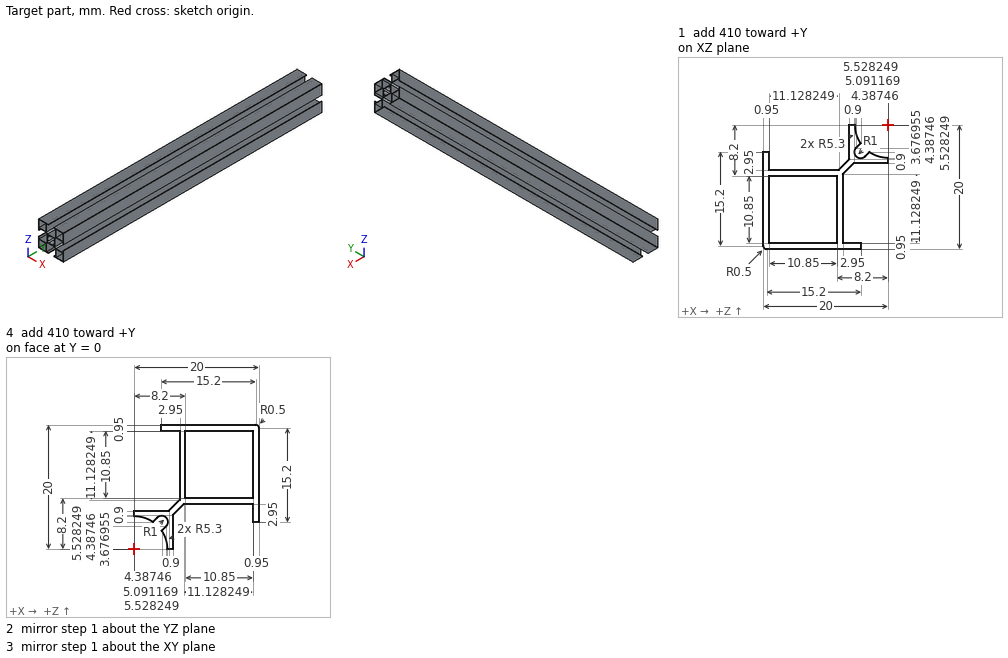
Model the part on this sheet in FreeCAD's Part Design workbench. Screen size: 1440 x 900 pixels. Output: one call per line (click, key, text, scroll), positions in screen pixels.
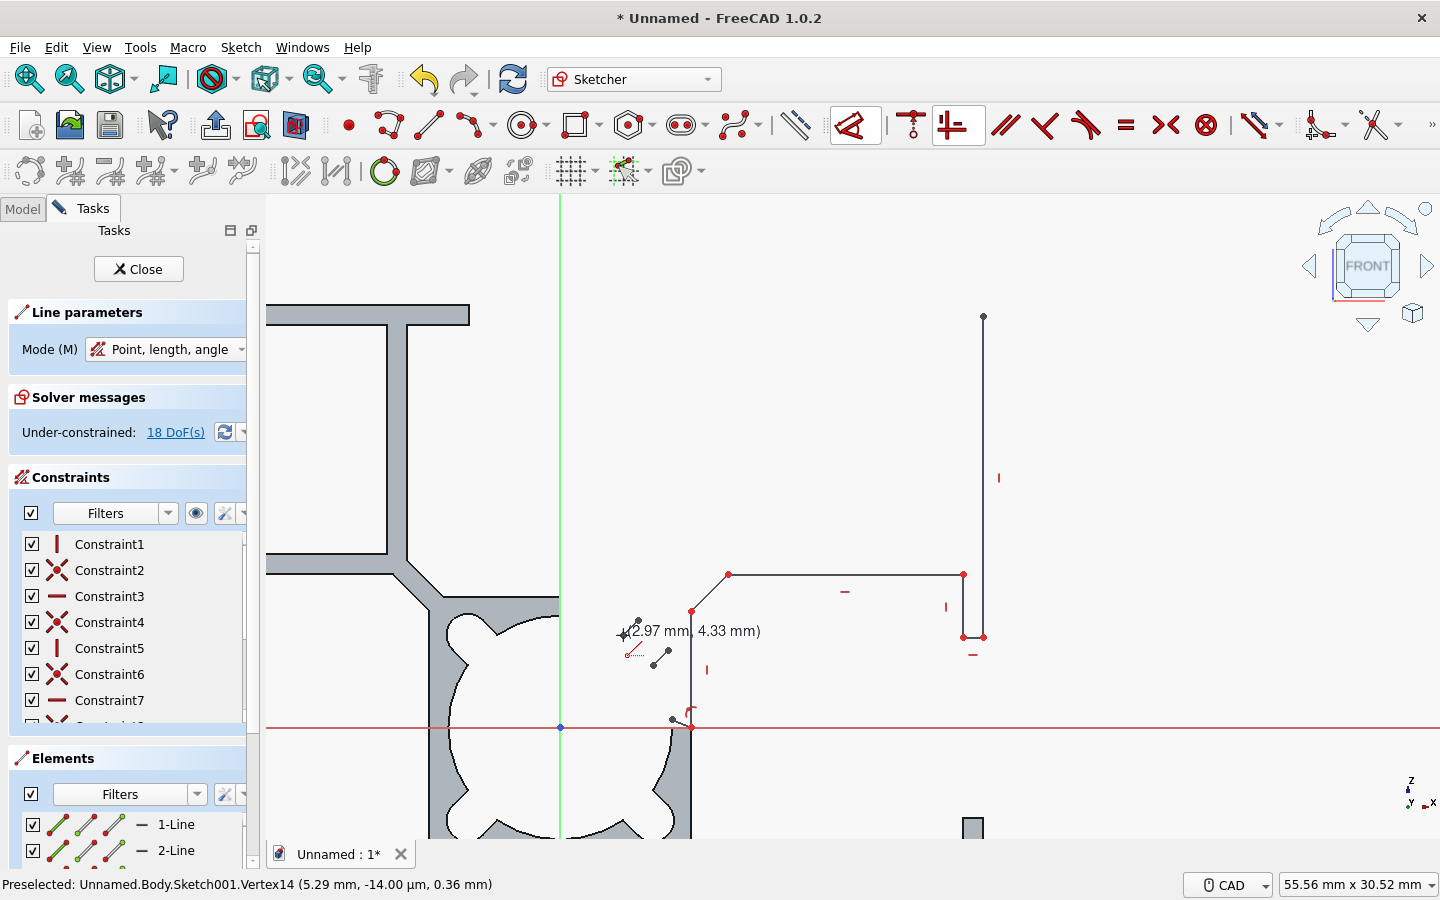
key(g)
key(m)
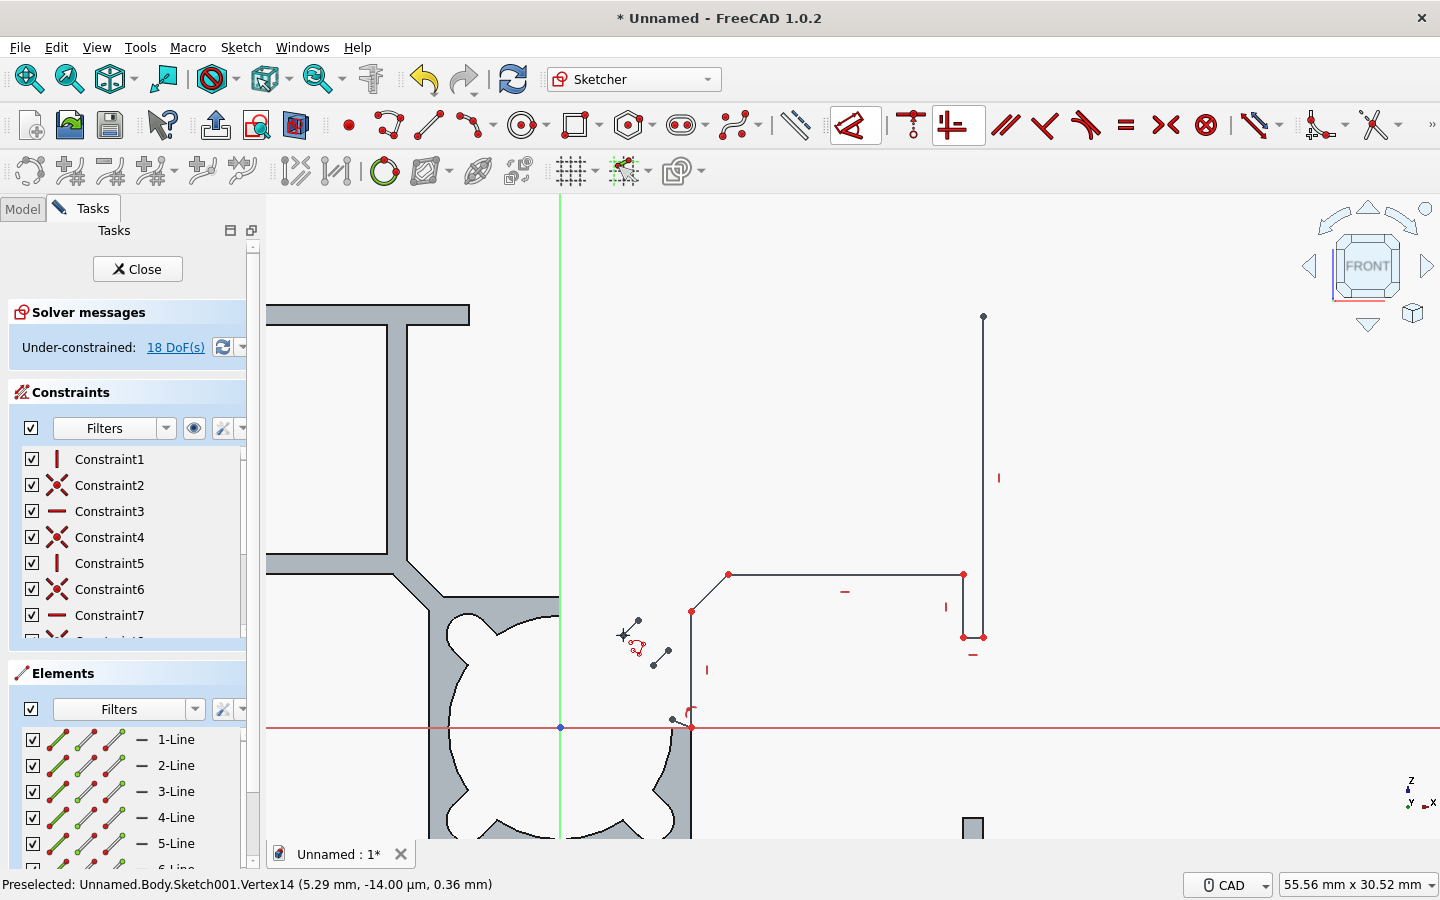
click(560, 616)
click(569, 597)
click(677, 597)
click(714, 560)
click(714, 325)
click(651, 325)
click(651, 305)
click(972, 305)
right_click(972, 305)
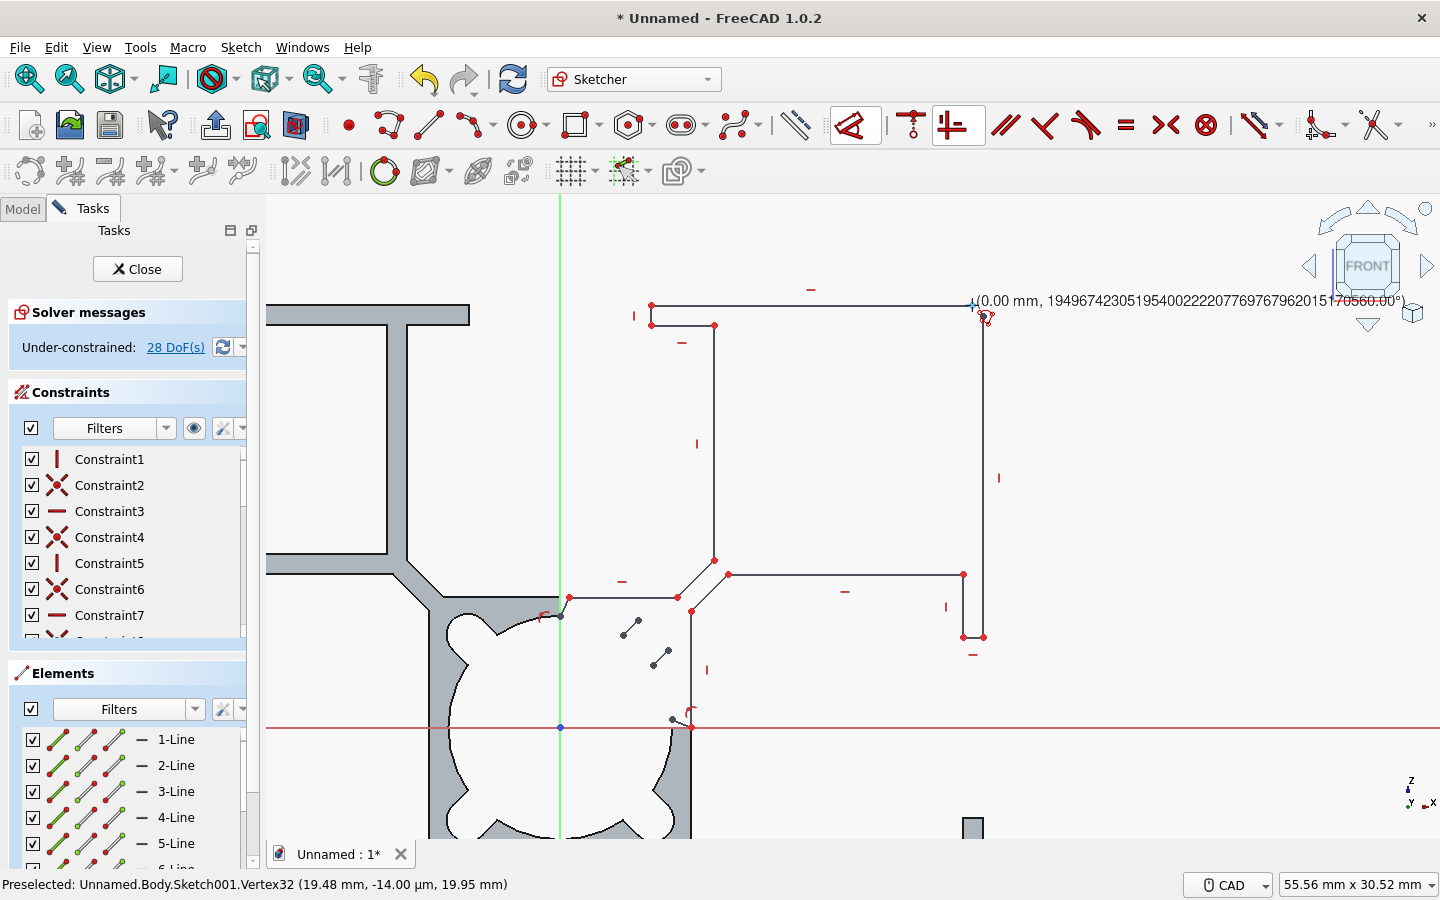
click(470, 126)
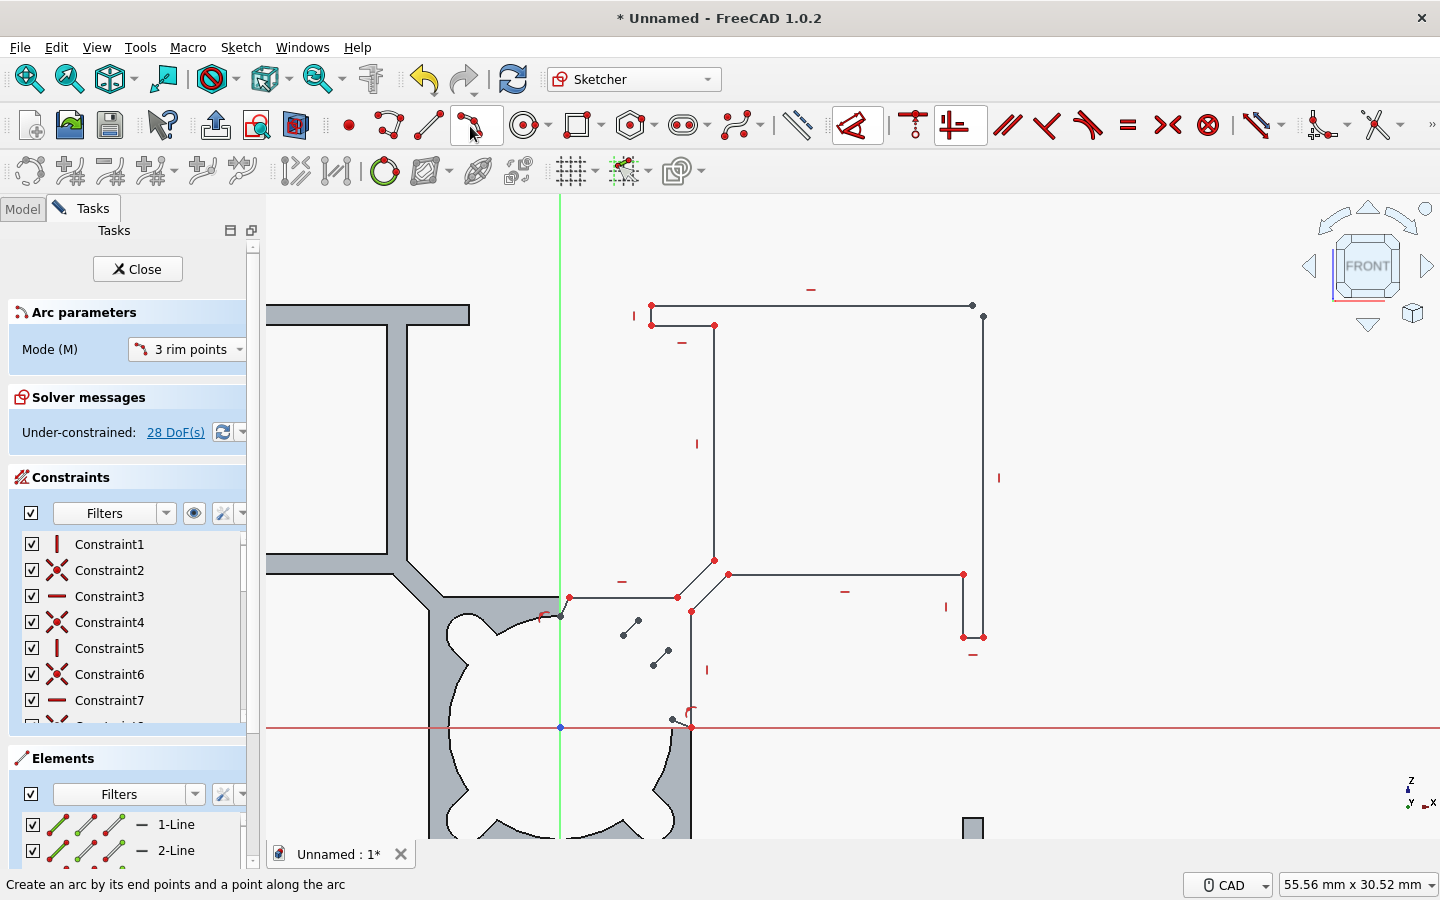
scroll(672, 728, up, 3)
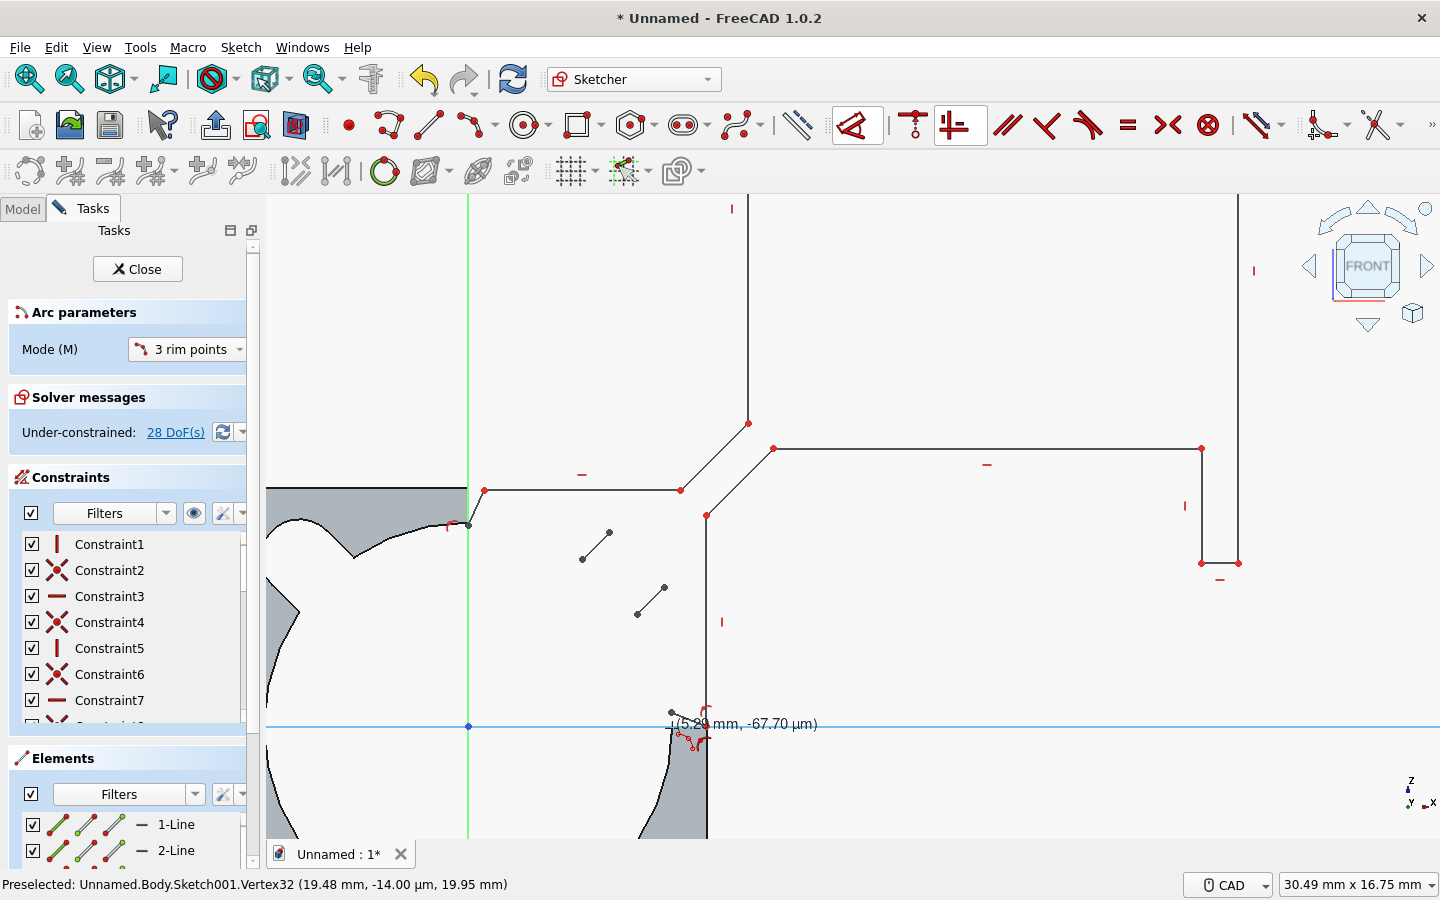
click(672, 713)
click(637, 614)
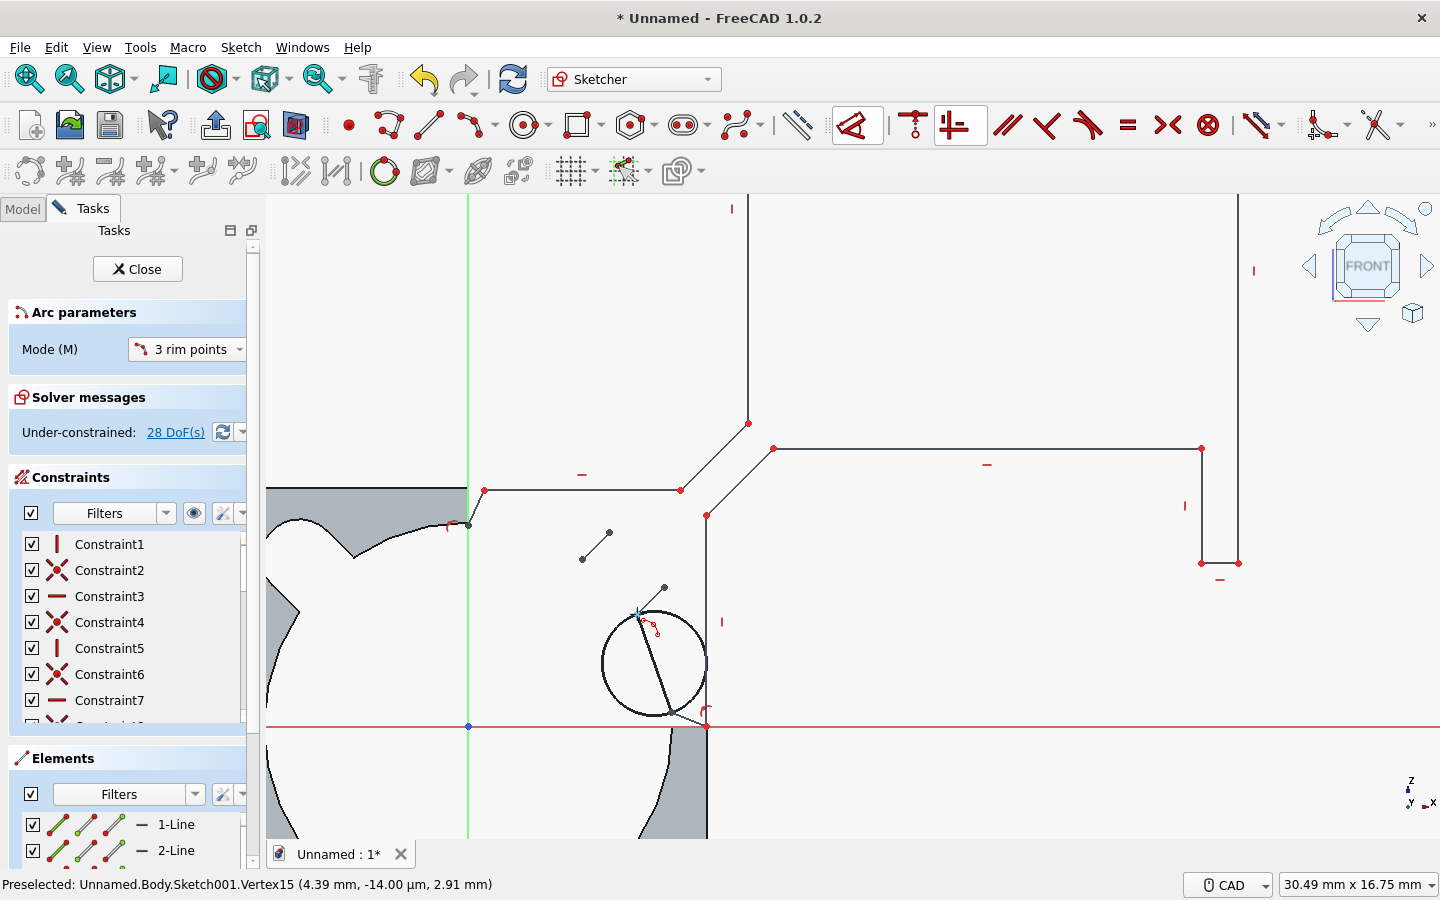
scroll(663, 667, up, 3)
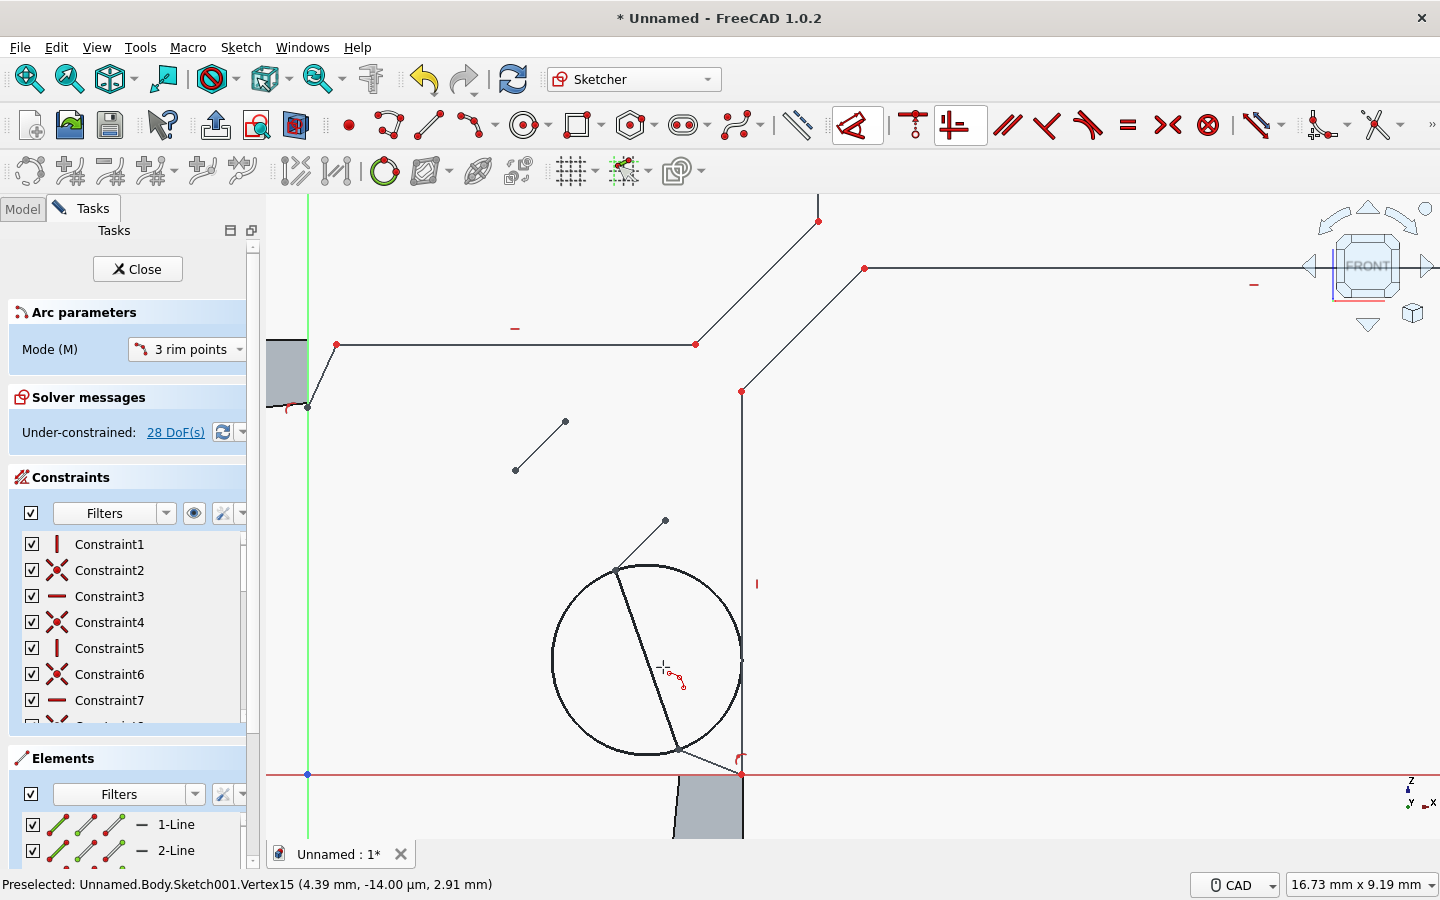
click(663, 666)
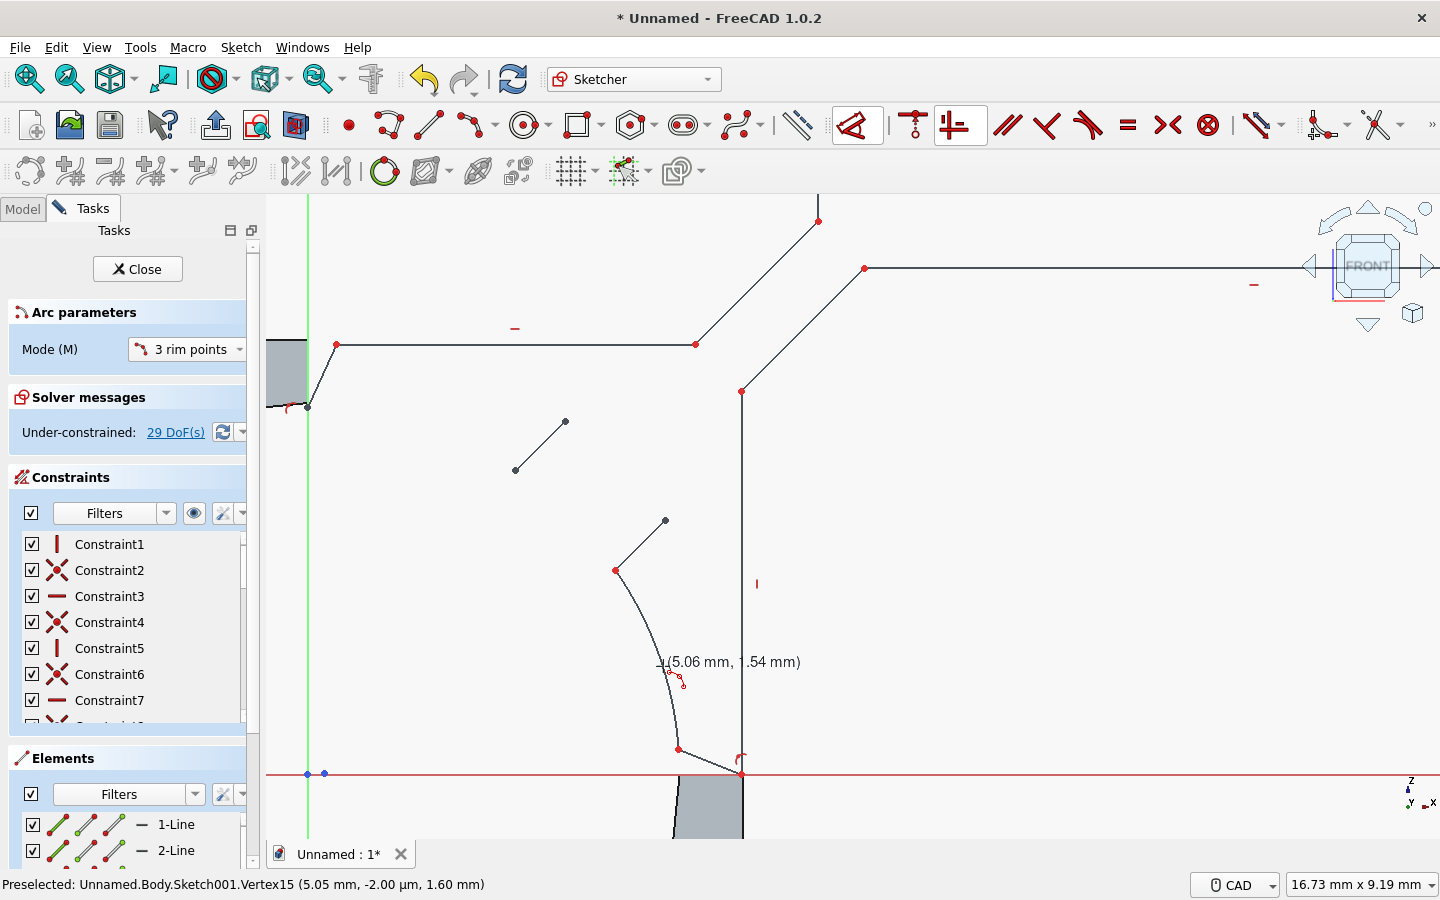
click(665, 521)
click(566, 421)
click(665, 418)